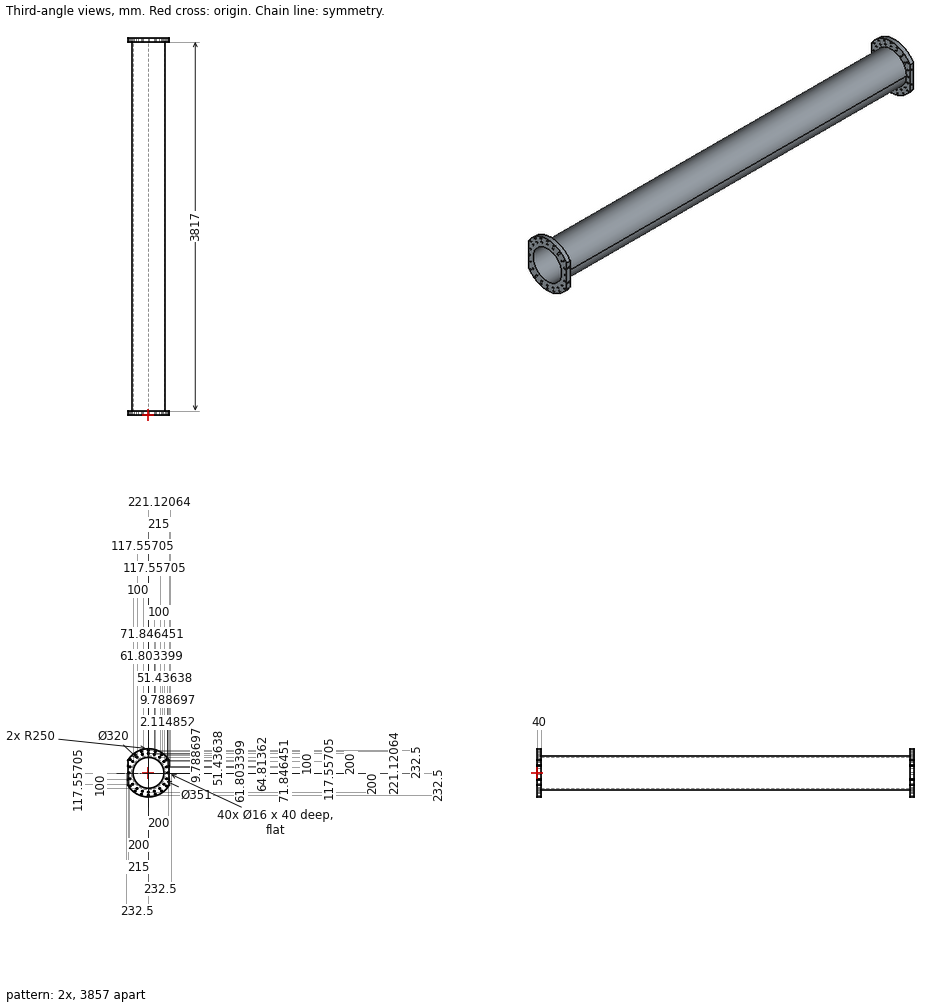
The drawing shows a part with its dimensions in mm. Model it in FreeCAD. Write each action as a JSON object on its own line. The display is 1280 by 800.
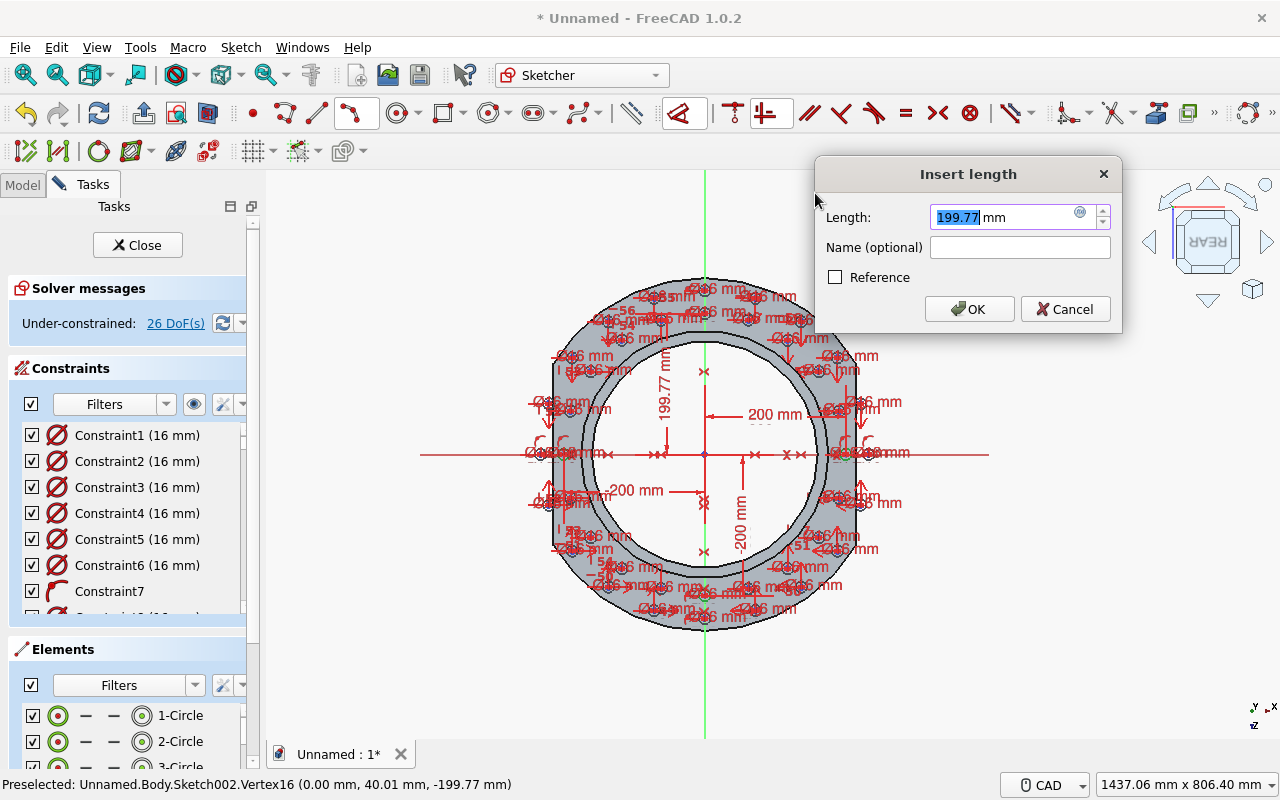
{"action": "type", "text": "200"}
{"action": "key", "text": "Return"}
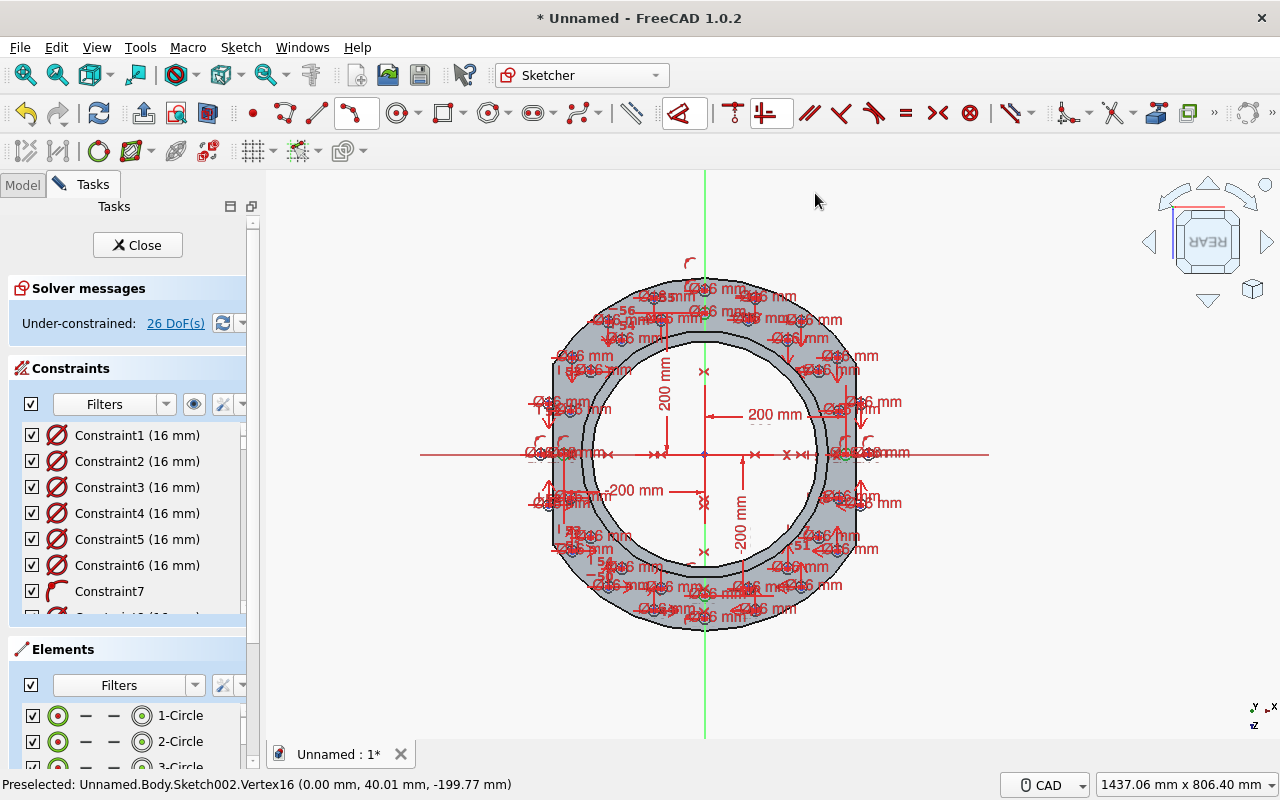
{"action": "left_click", "coordinate": [839, 498]}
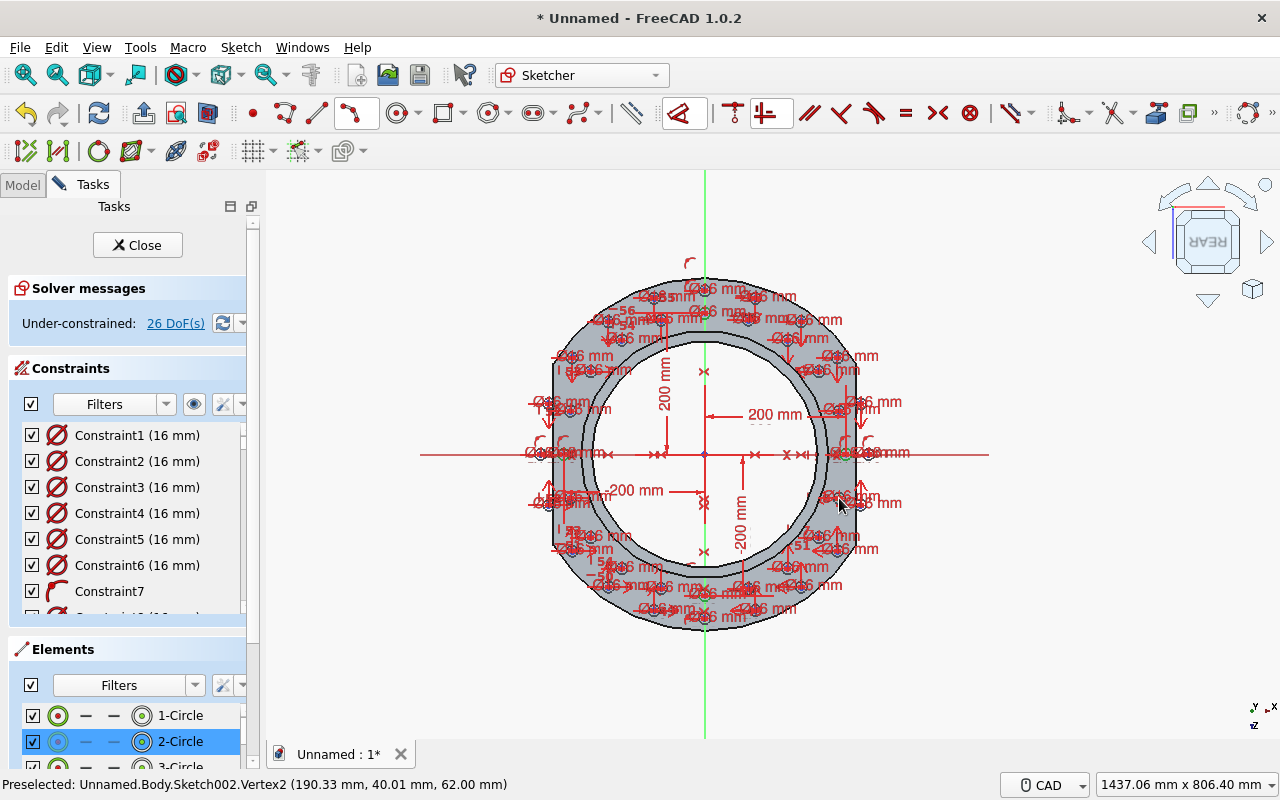
{"action": "left_click", "coordinate": [788, 569]}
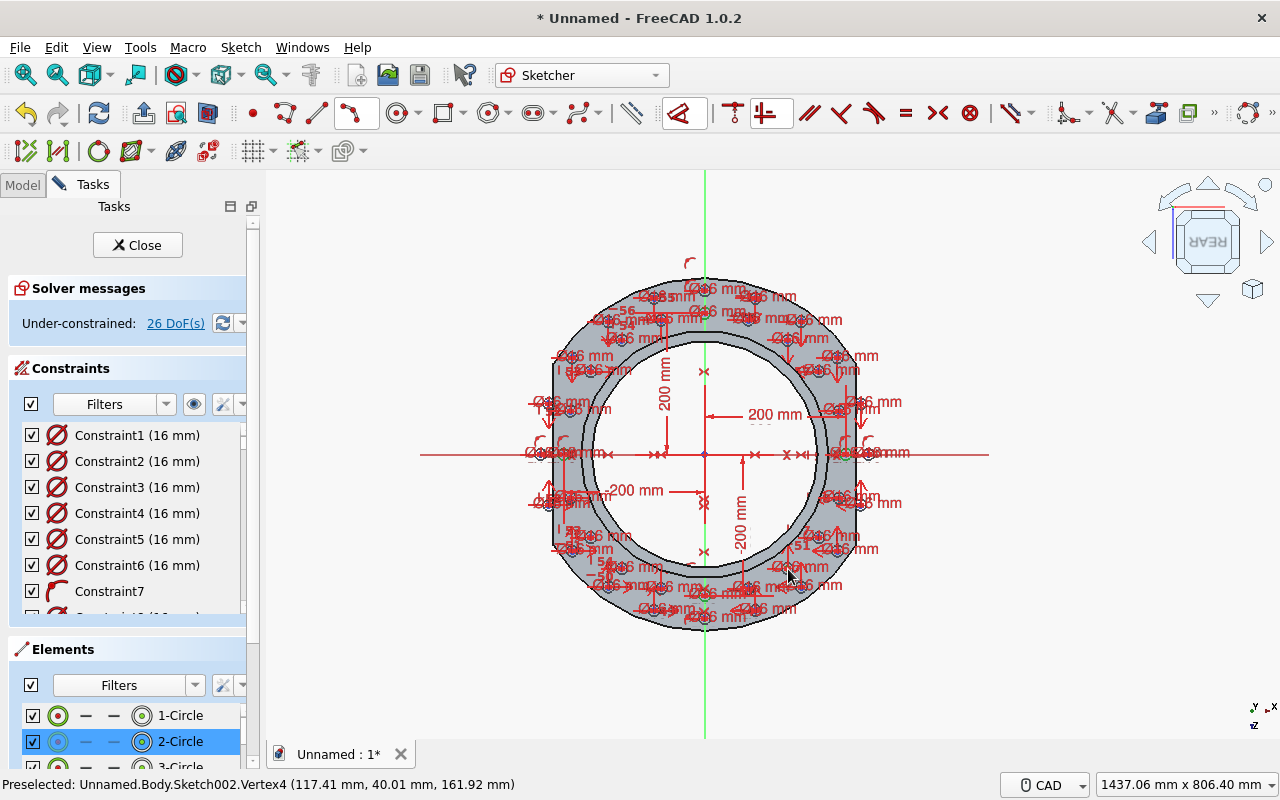
{"action": "left_click", "coordinate": [702, 114]}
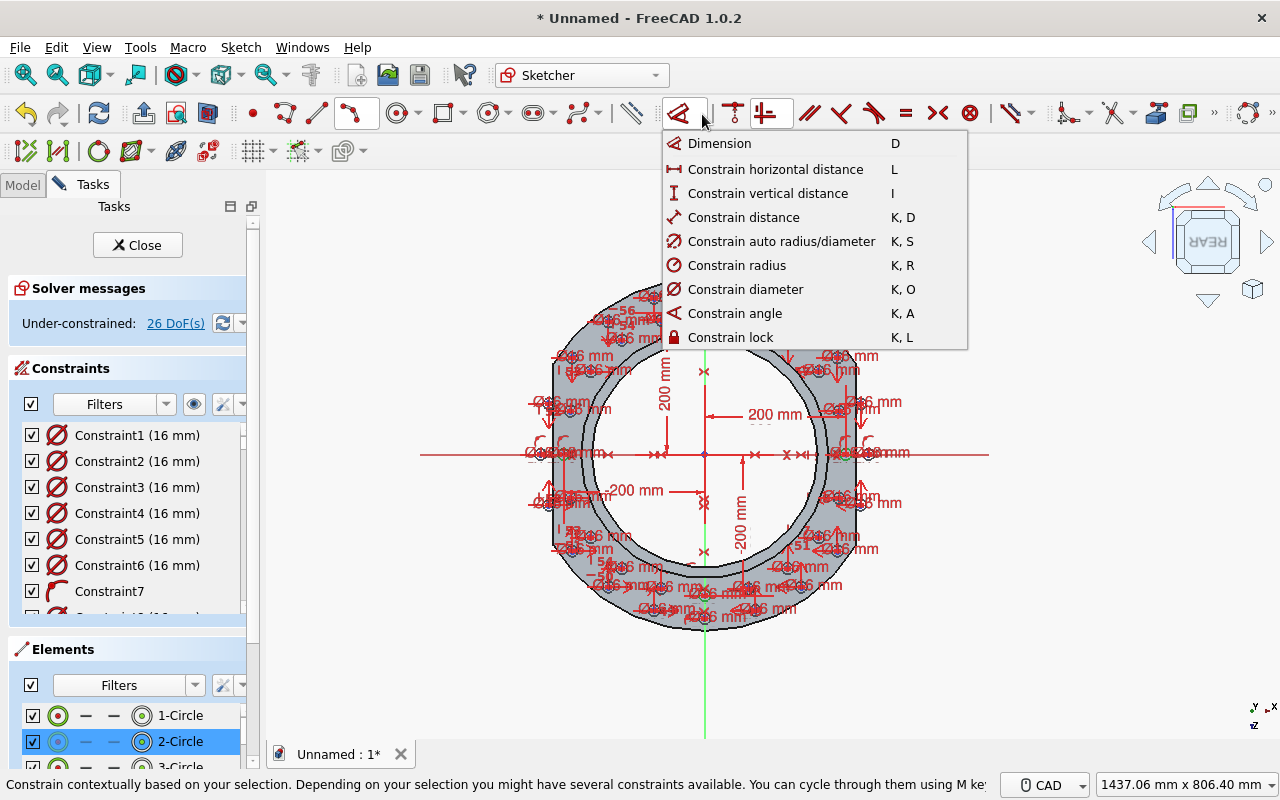
{"action": "left_click", "coordinate": [815, 193]}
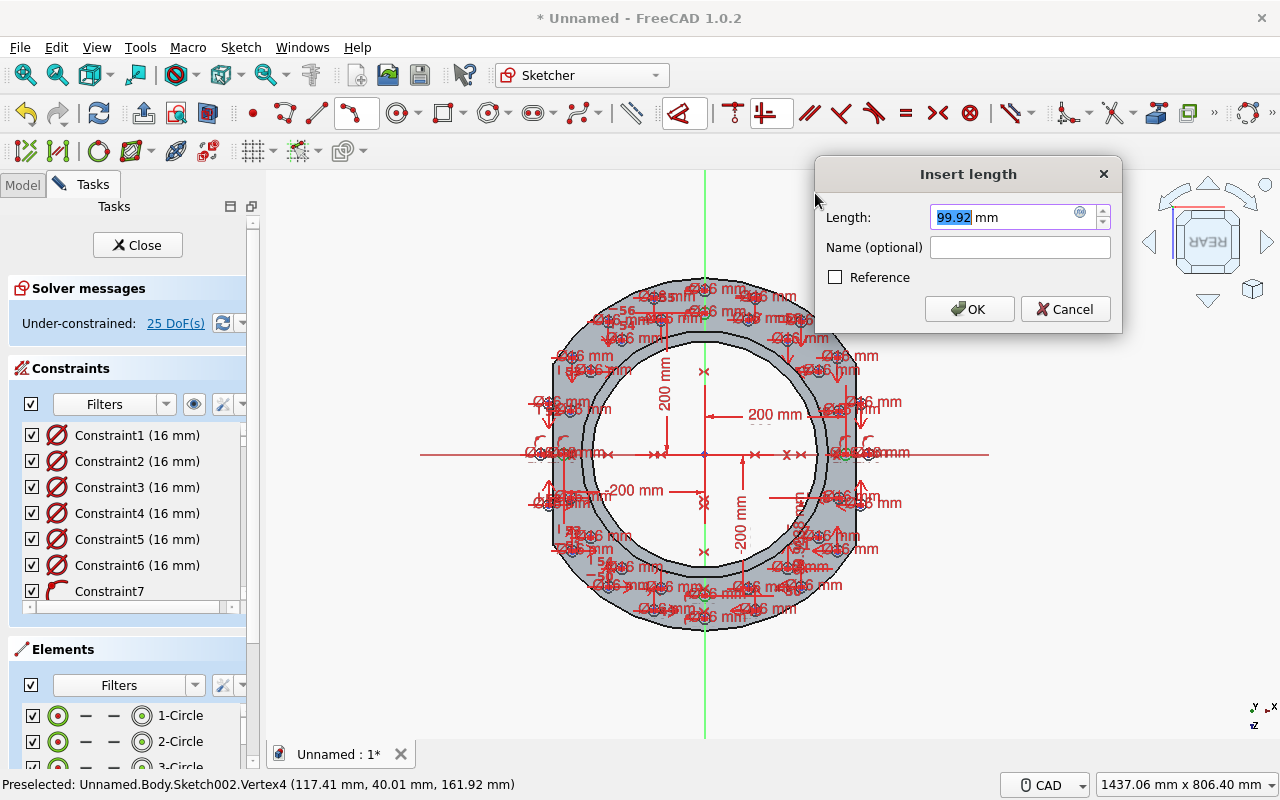
{"action": "type", "text": "100"}
{"action": "key", "text": "Return"}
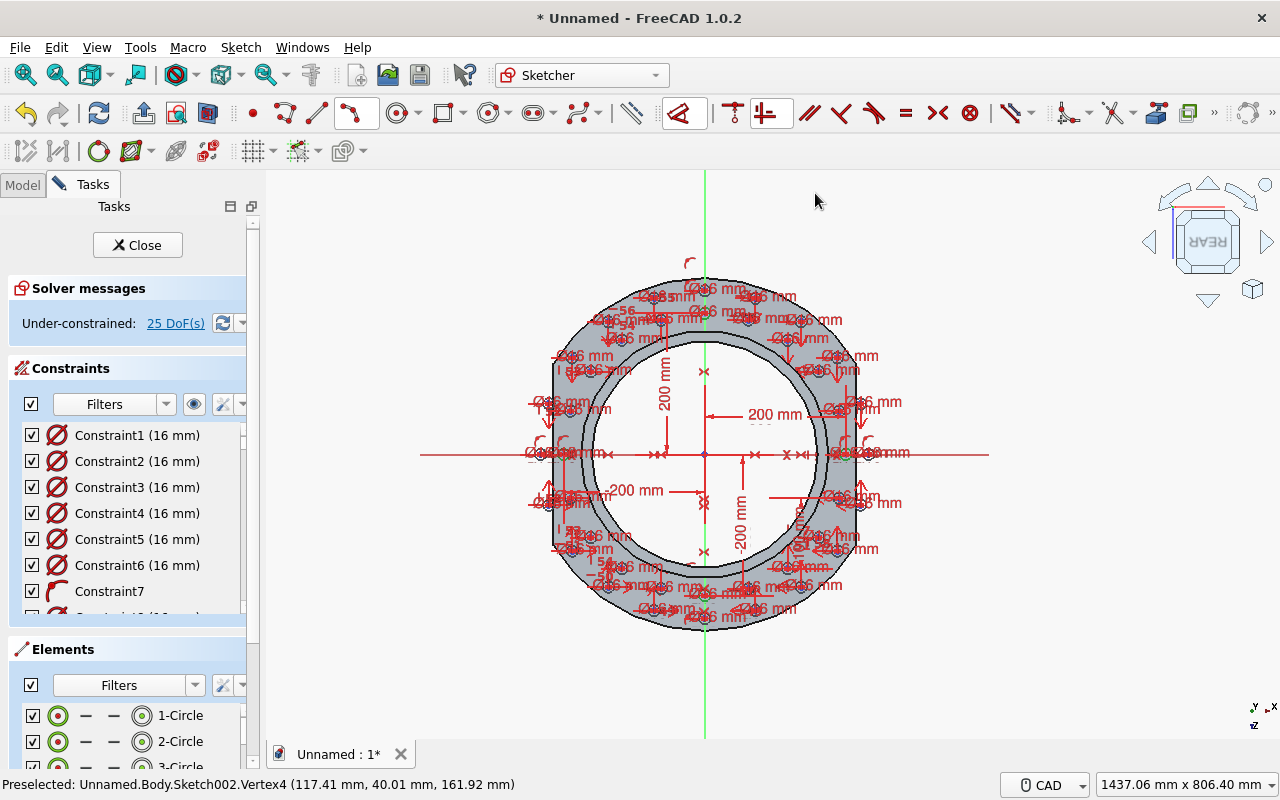
{"action": "left_click", "coordinate": [819, 538]}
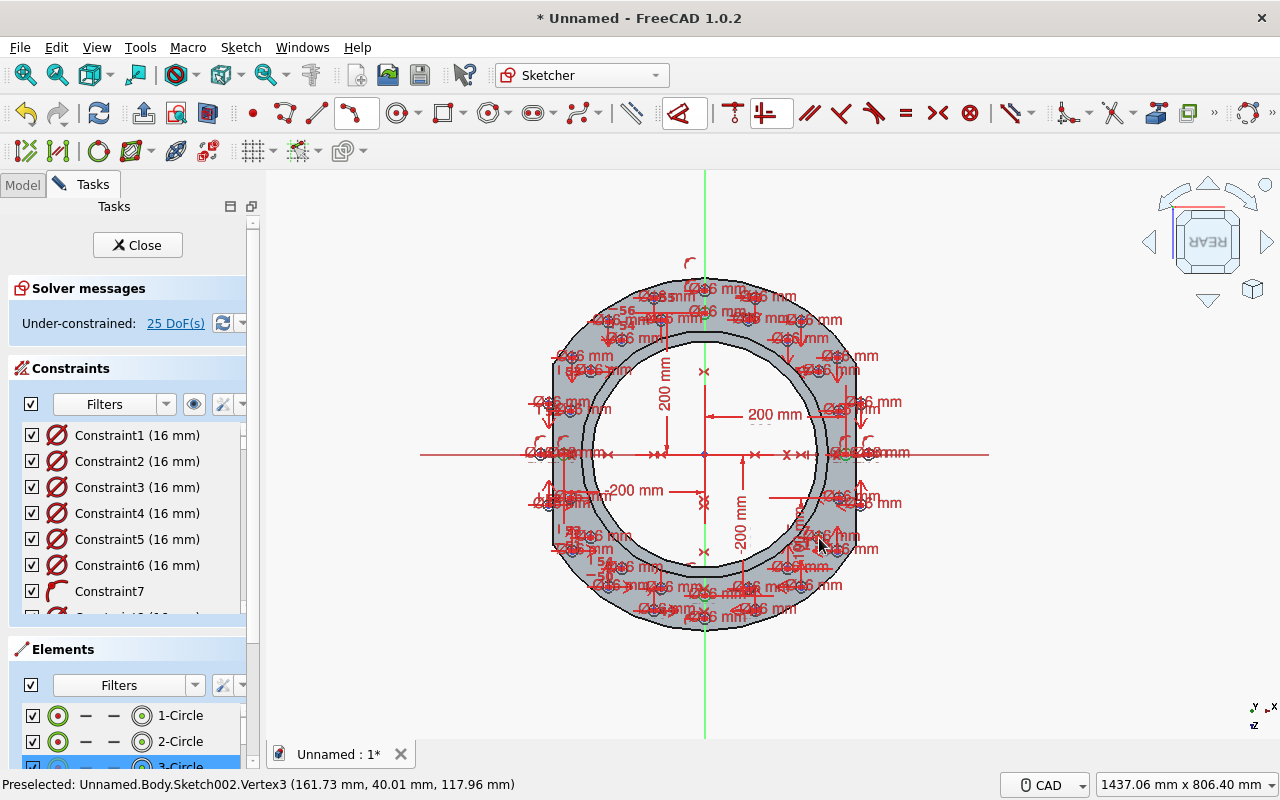
{"action": "left_click", "coordinate": [748, 589]}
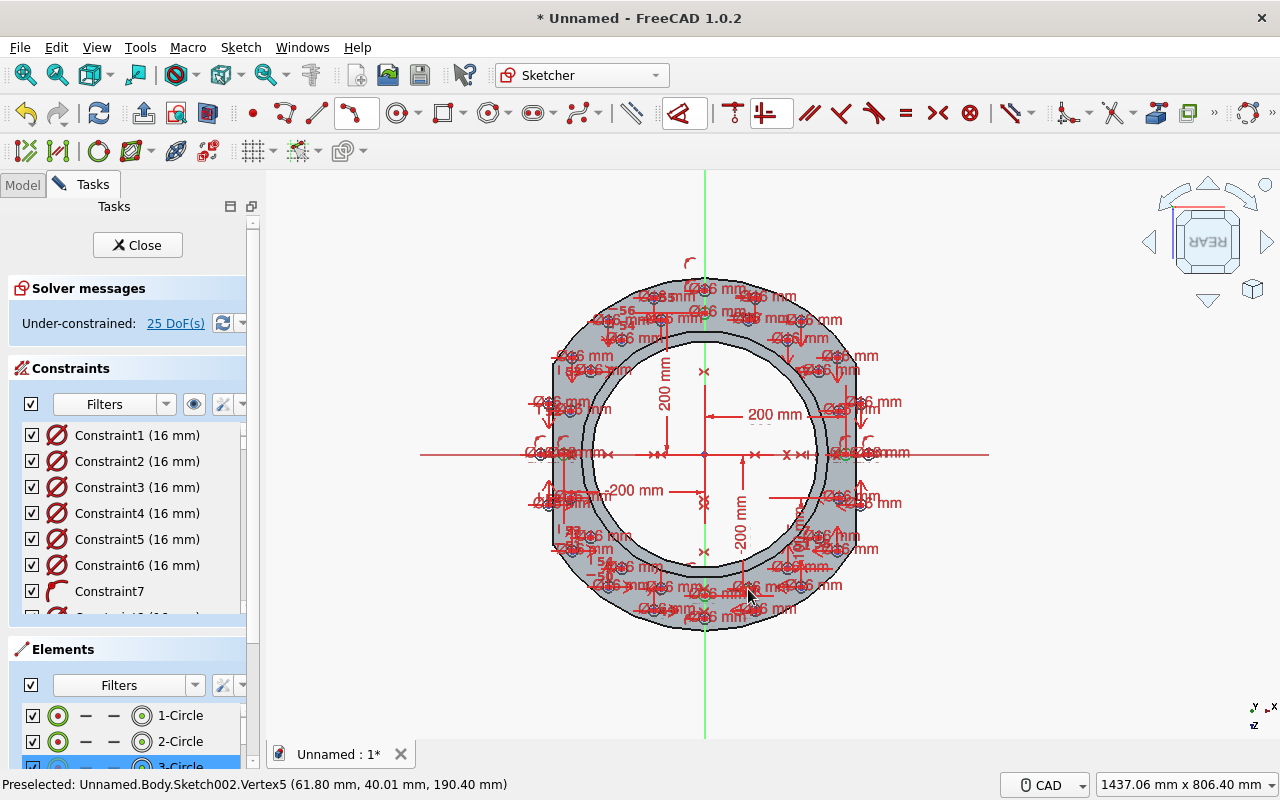
{"action": "left_click", "coordinate": [702, 114]}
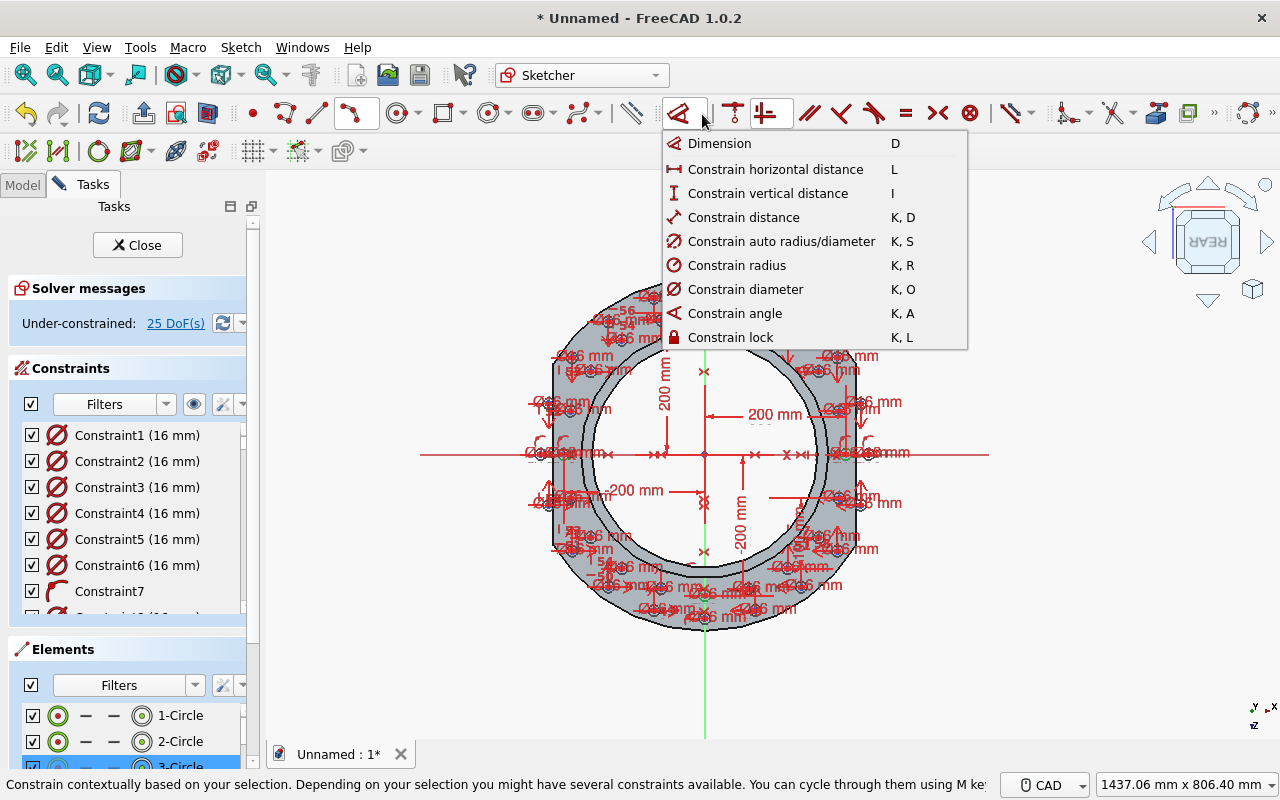
{"action": "left_click", "coordinate": [815, 169]}